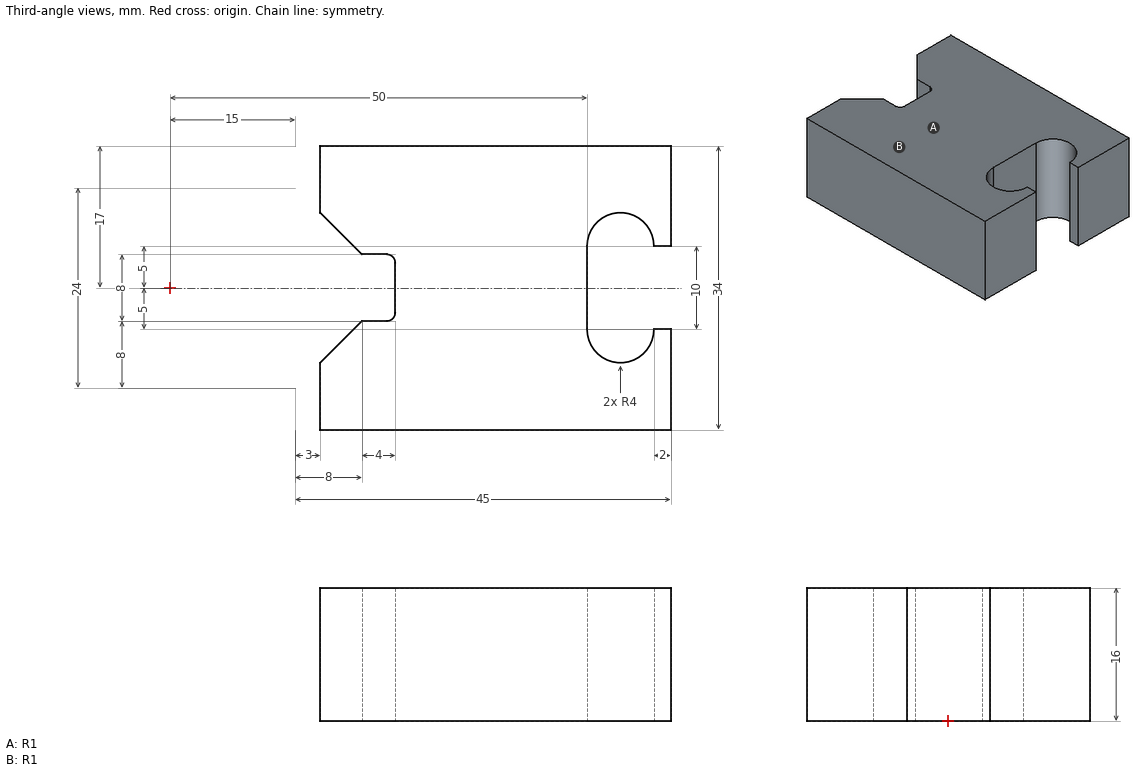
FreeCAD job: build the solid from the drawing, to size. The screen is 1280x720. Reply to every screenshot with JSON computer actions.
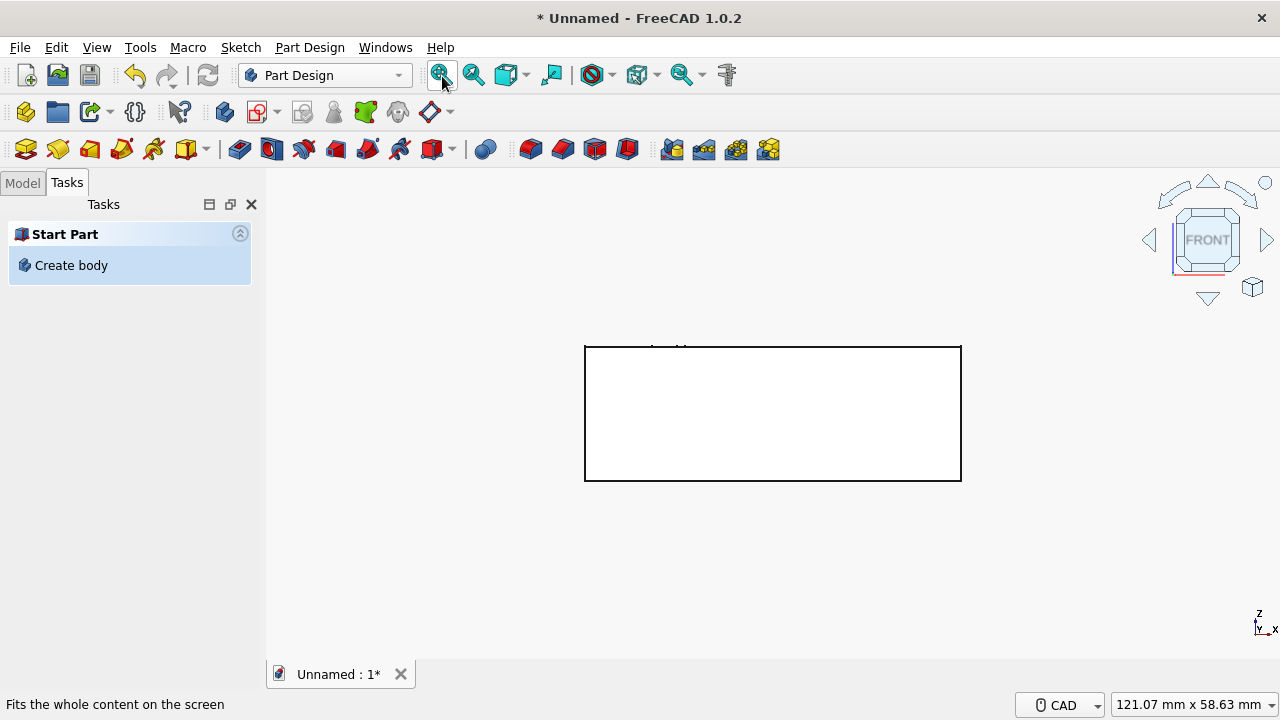
{"action": "key", "text": "3"}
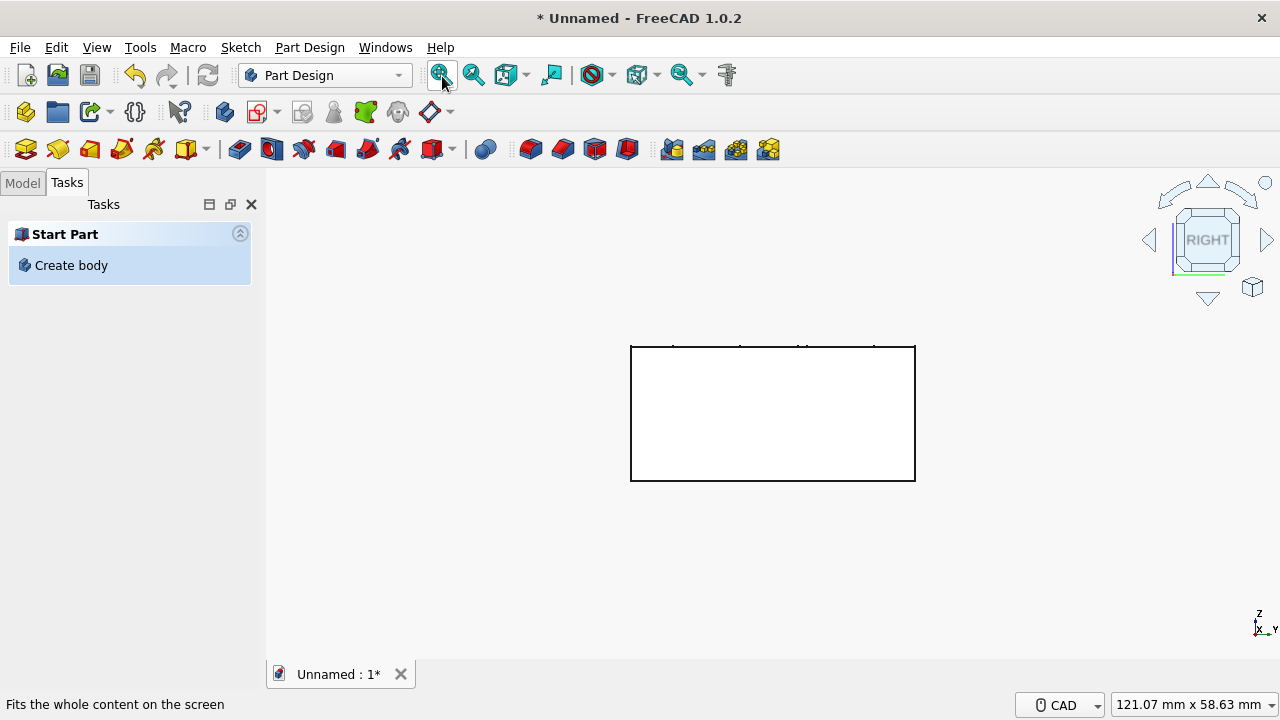
{"action": "left_click", "coordinate": [442, 76]}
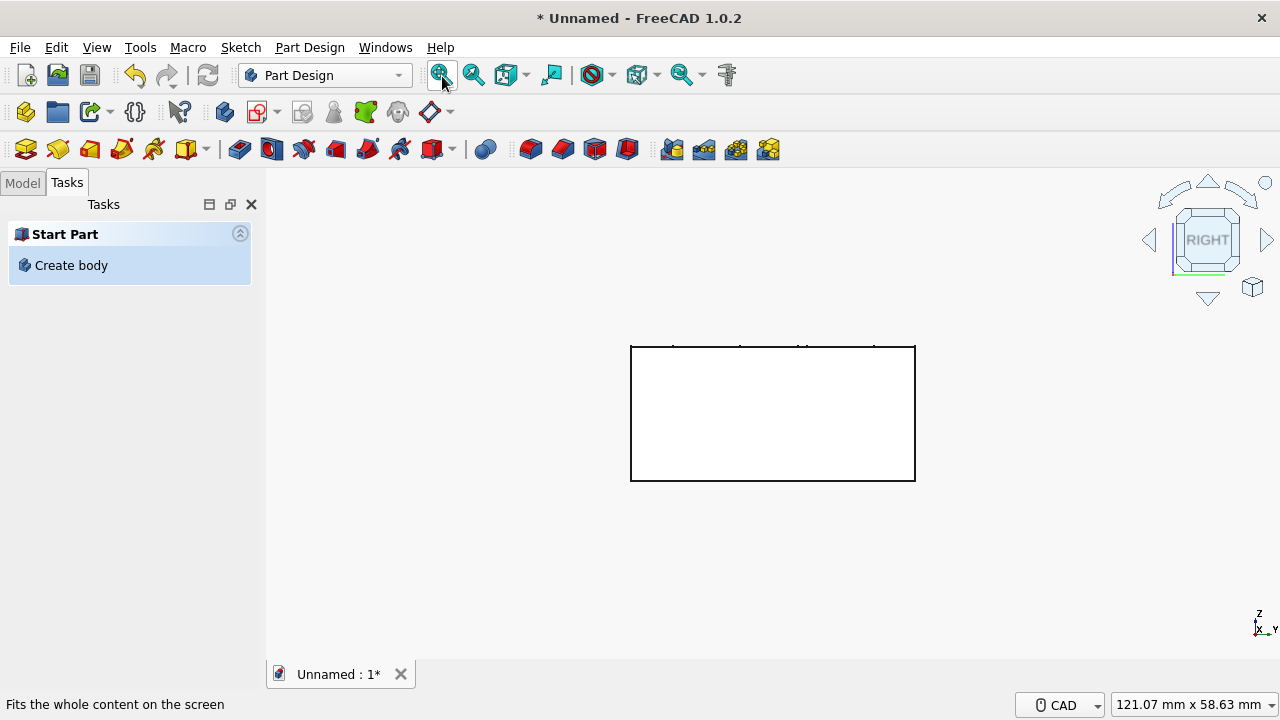
{"action": "key", "text": "5"}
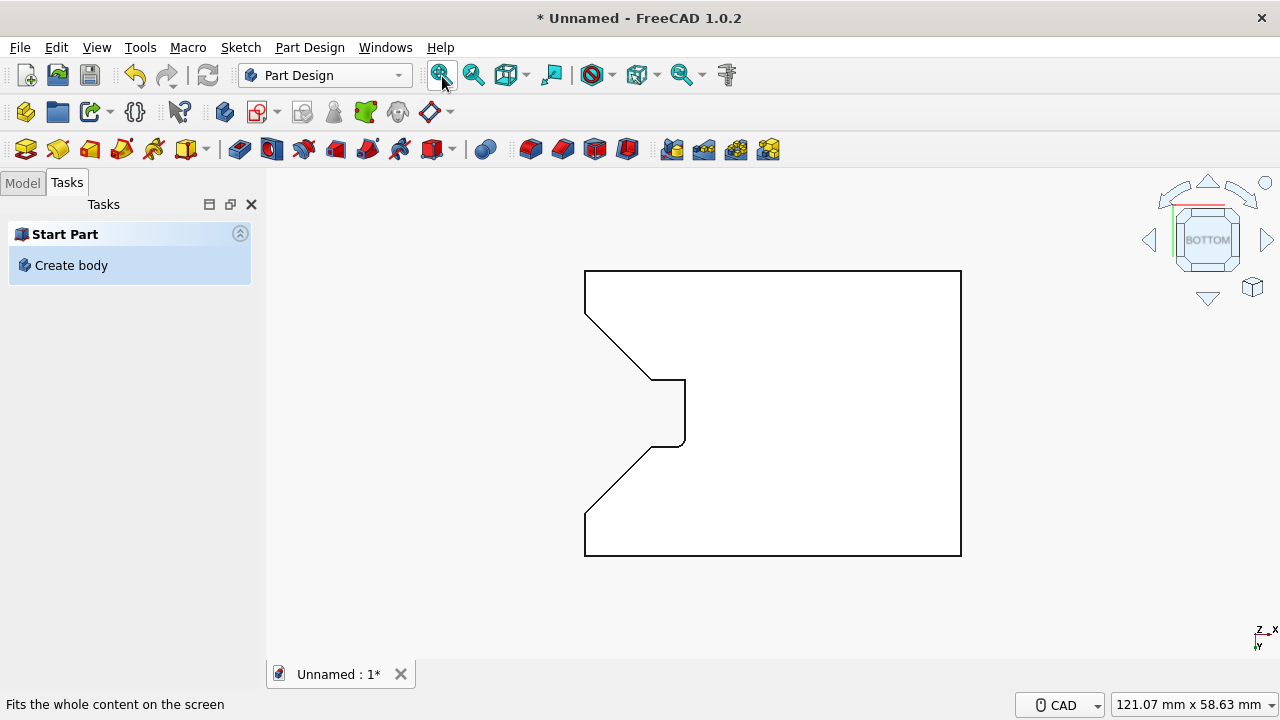
{"action": "key", "text": "4"}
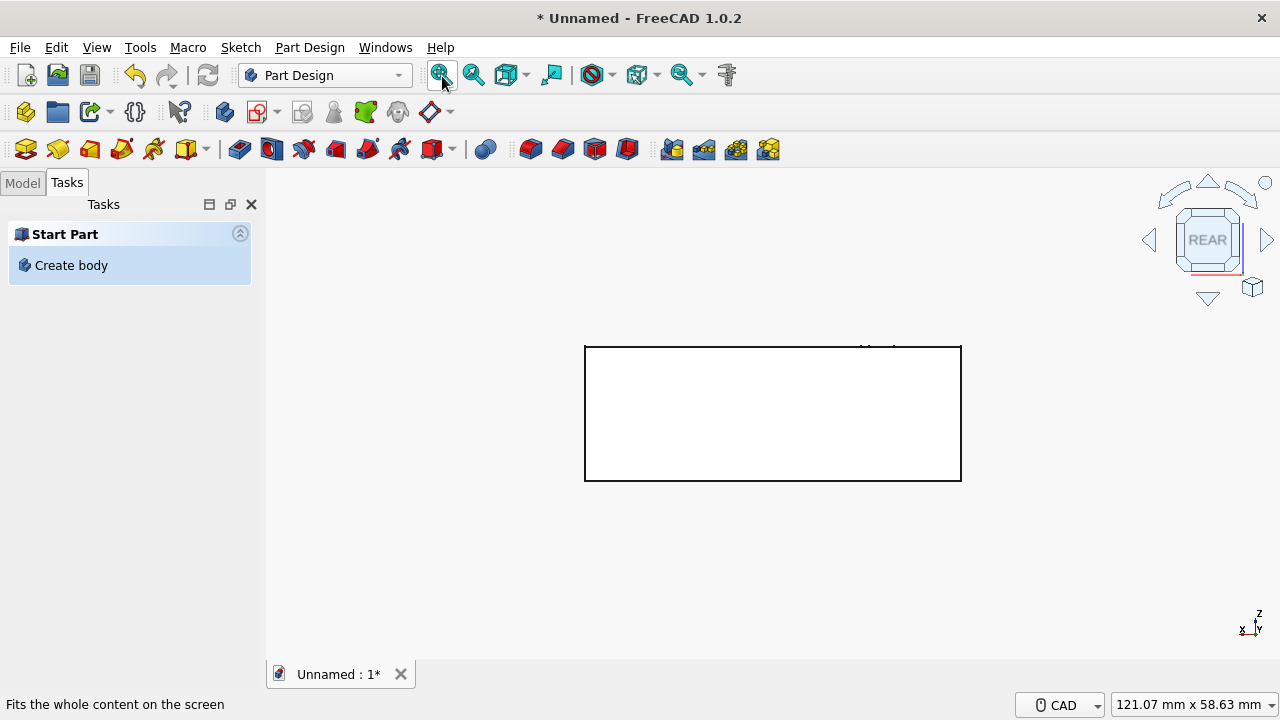
{"action": "left_click", "coordinate": [442, 76]}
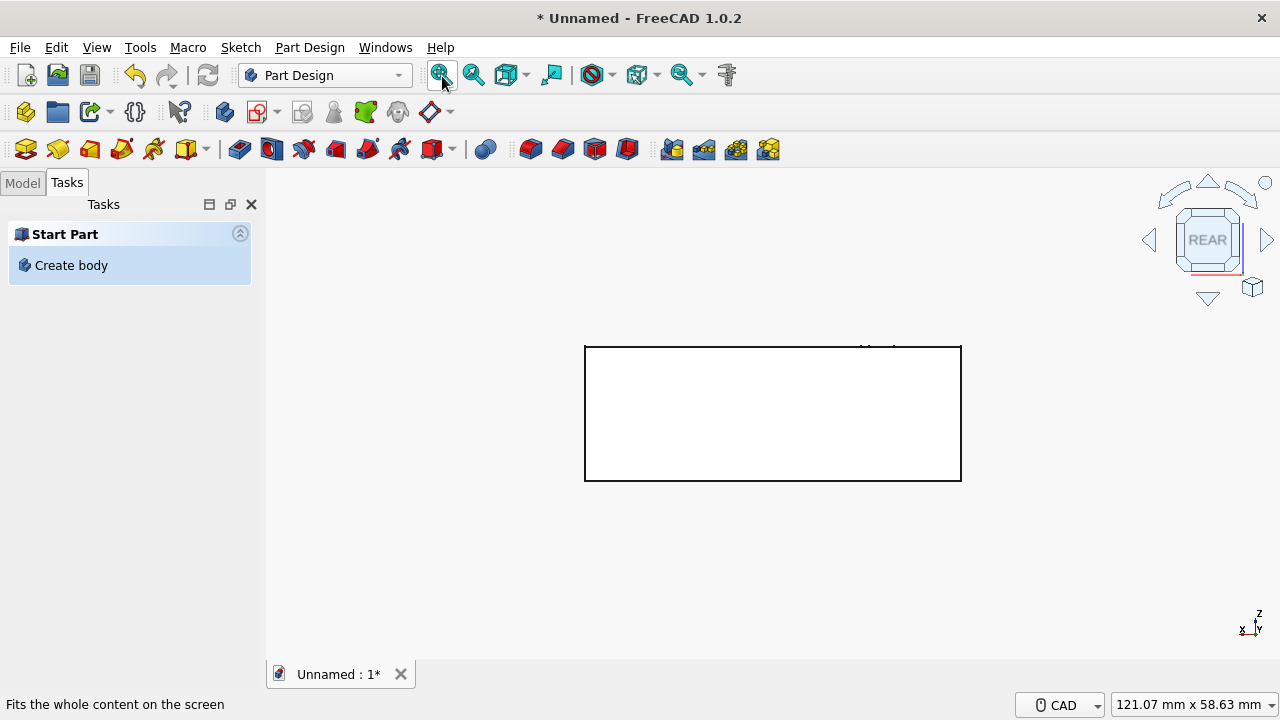
{"action": "key", "text": "6"}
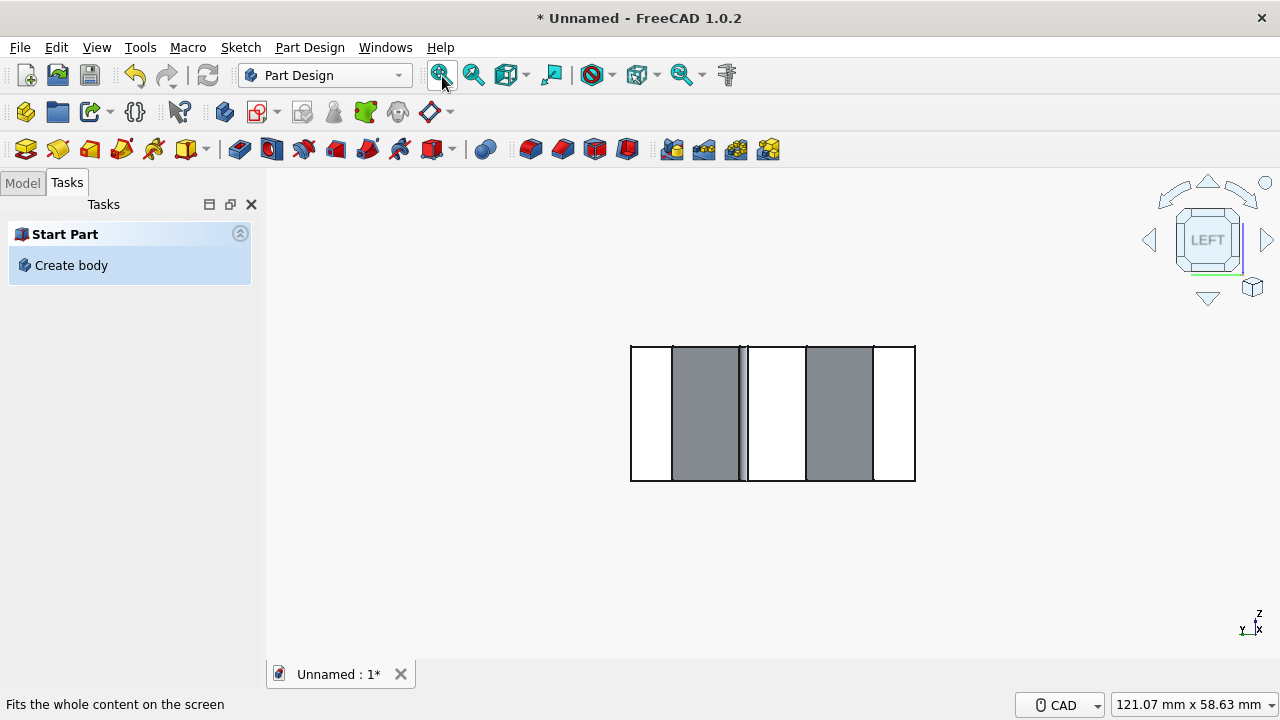
{"action": "left_click", "coordinate": [442, 76]}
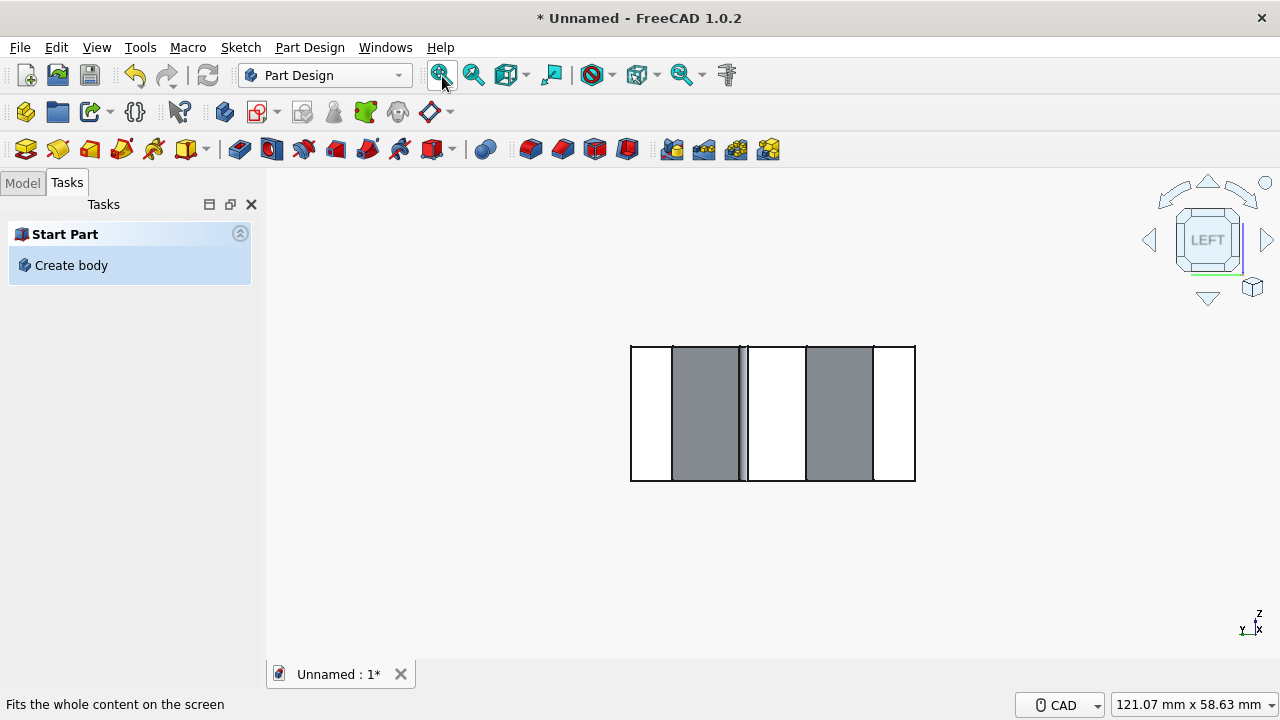
{"action": "key", "text": "v 3"}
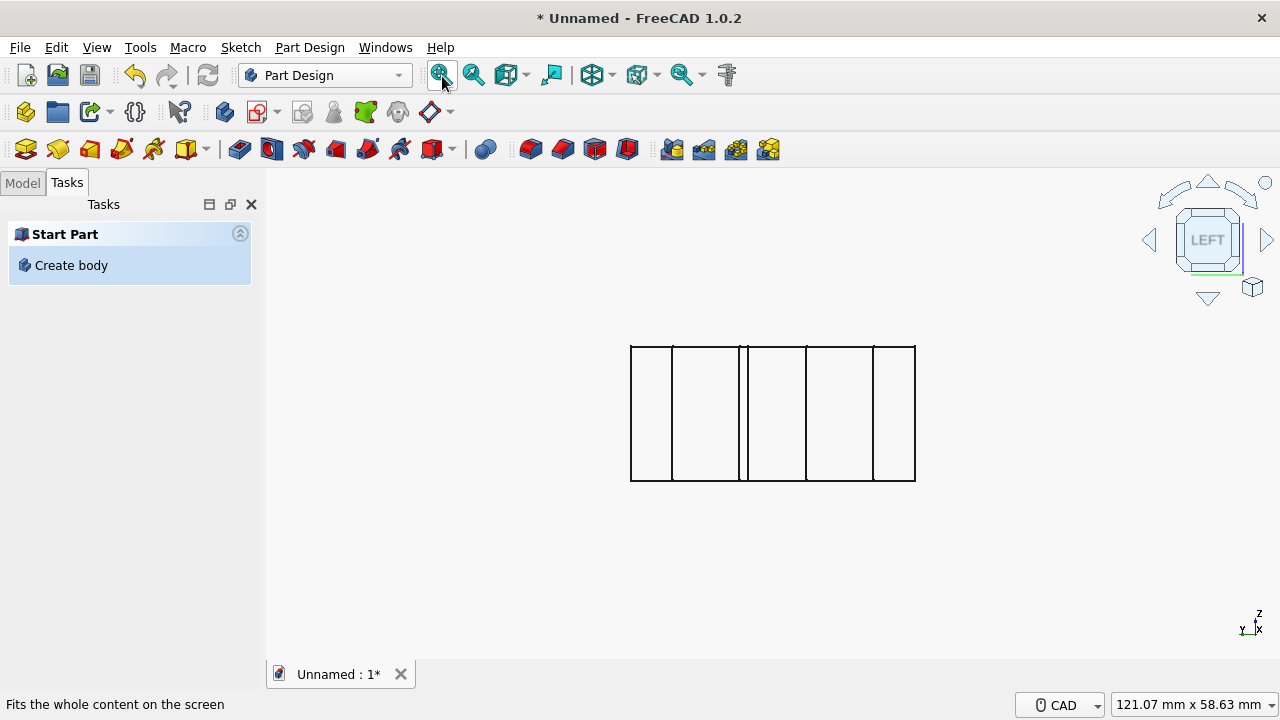
{"action": "key", "text": "0"}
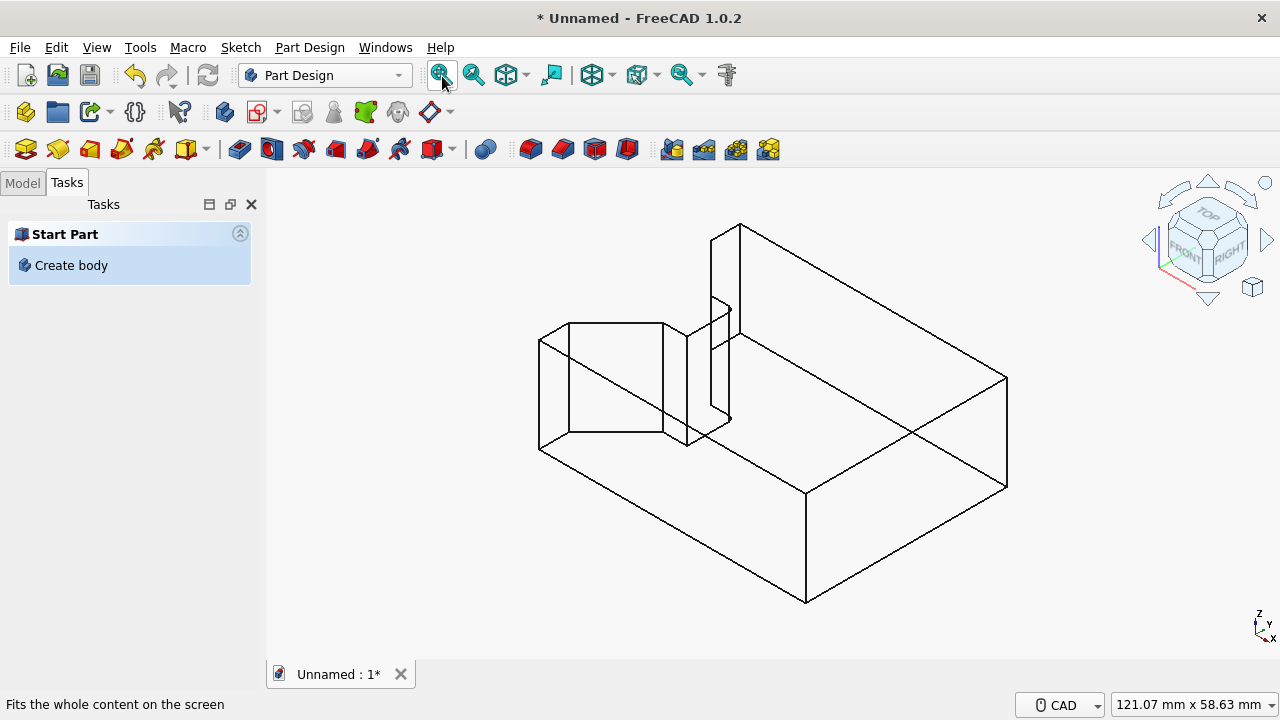
{"action": "left_click", "coordinate": [687, 390]}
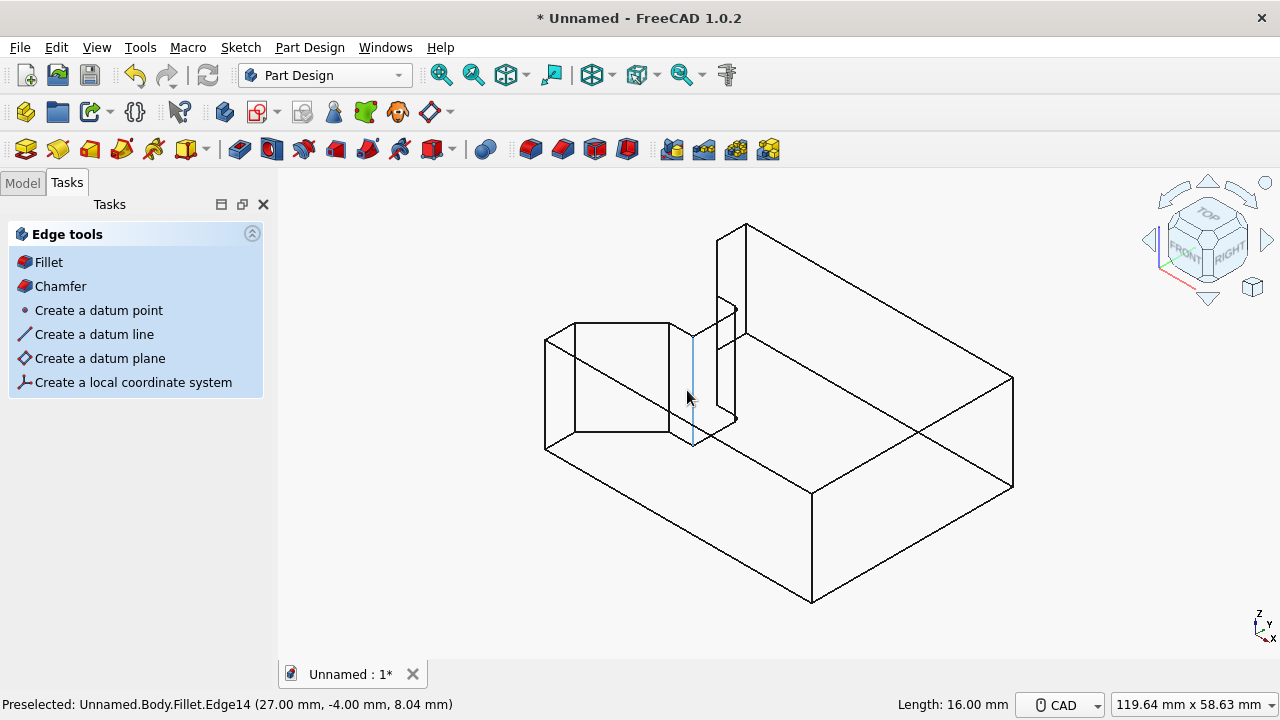
{"action": "key", "text": "v 1"}